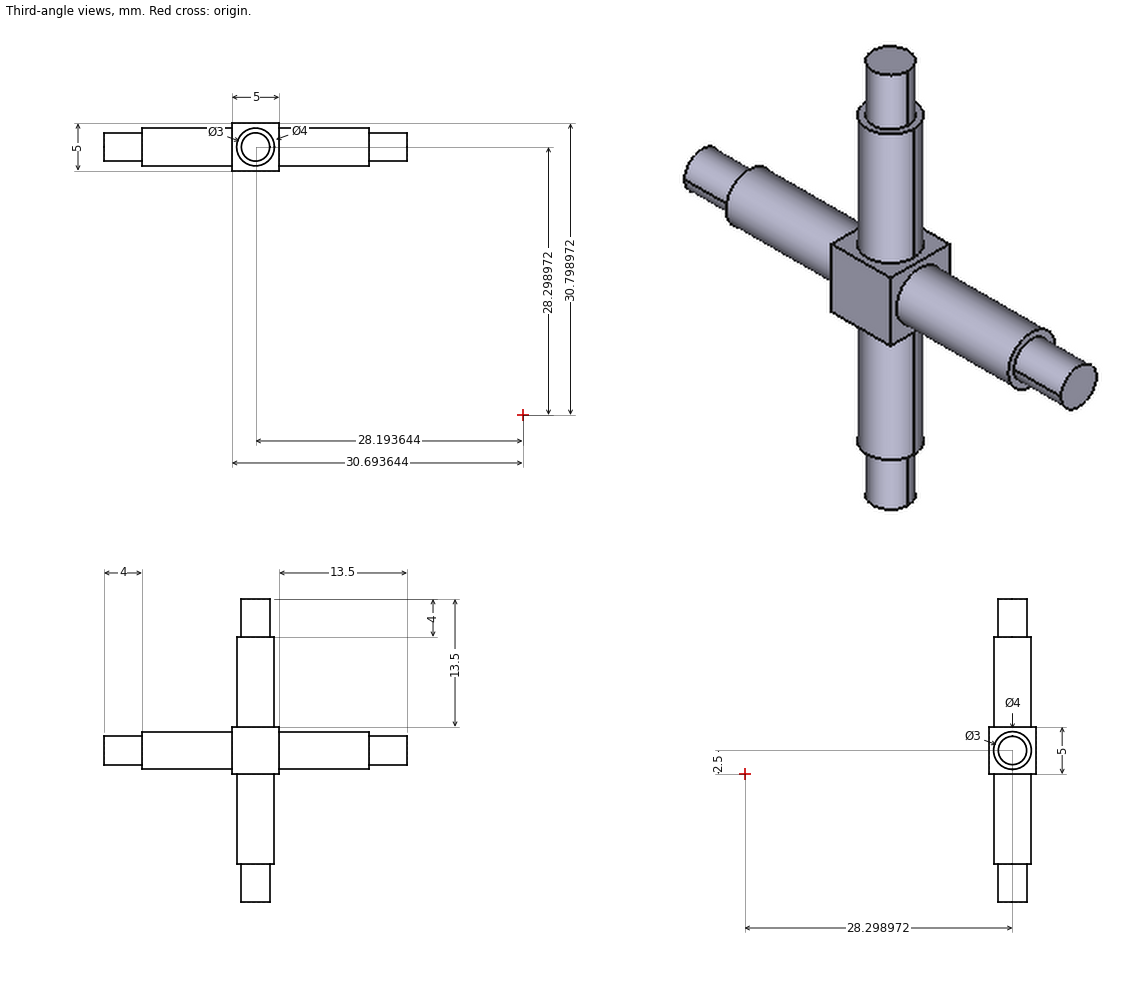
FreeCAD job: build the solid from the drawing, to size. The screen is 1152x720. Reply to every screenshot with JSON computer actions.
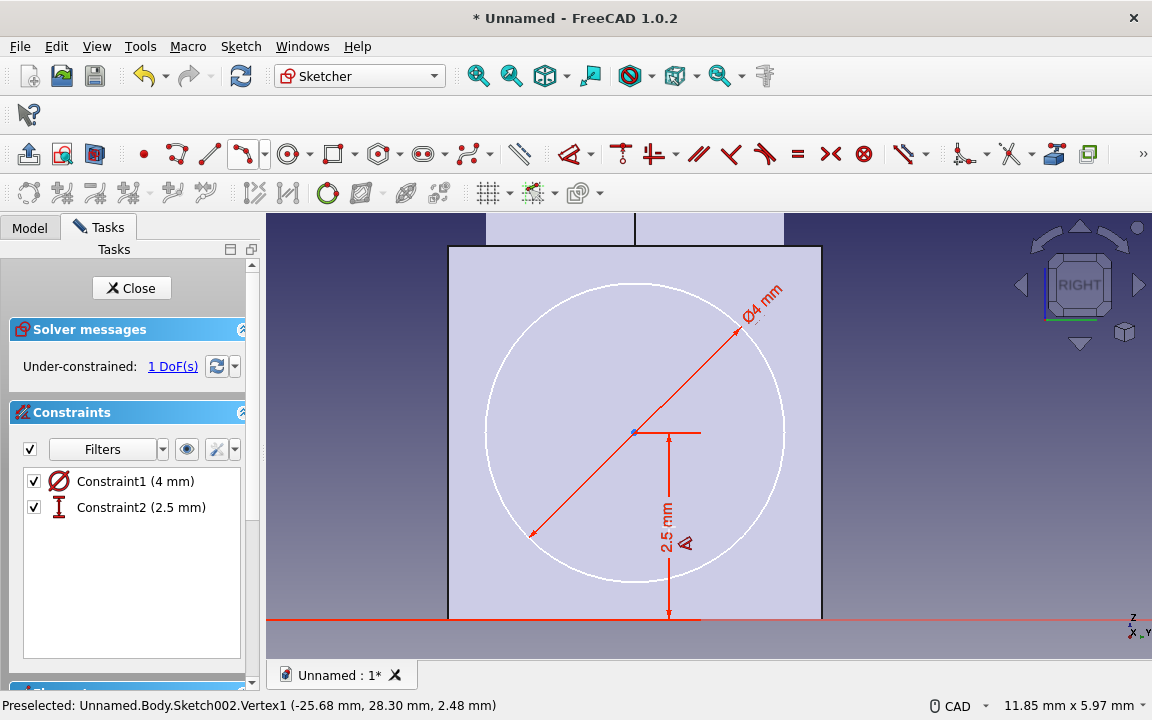
{"action": "left_click", "coordinate": [635, 433]}
{"action": "left_click", "coordinate": [464, 399]}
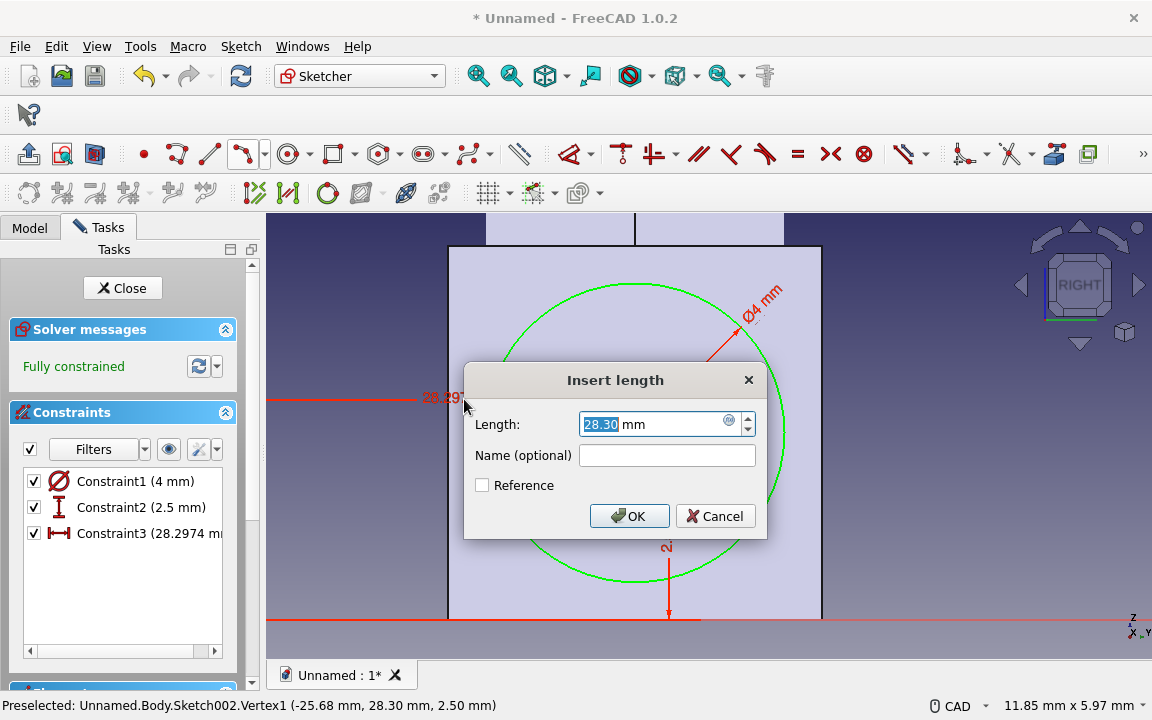
{"action": "type", "text": "28.298972"}
{"action": "key", "text": "Return"}
{"action": "key", "text": "Escape"}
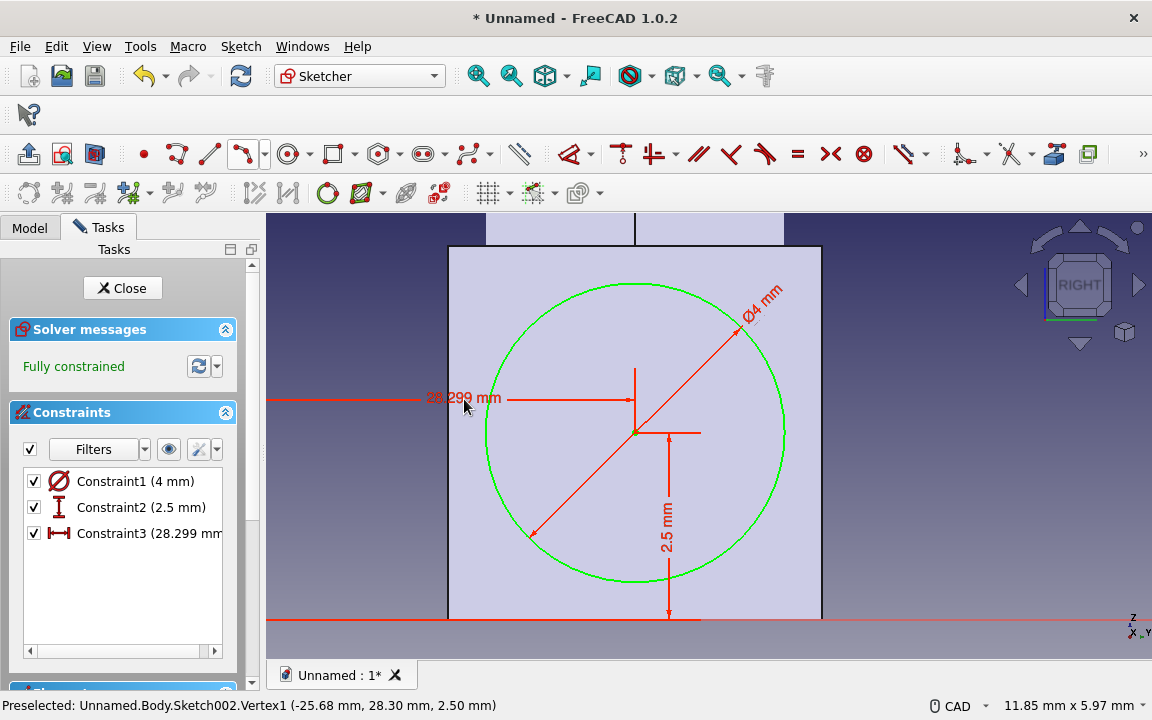
{"action": "left_click", "coordinate": [123, 288]}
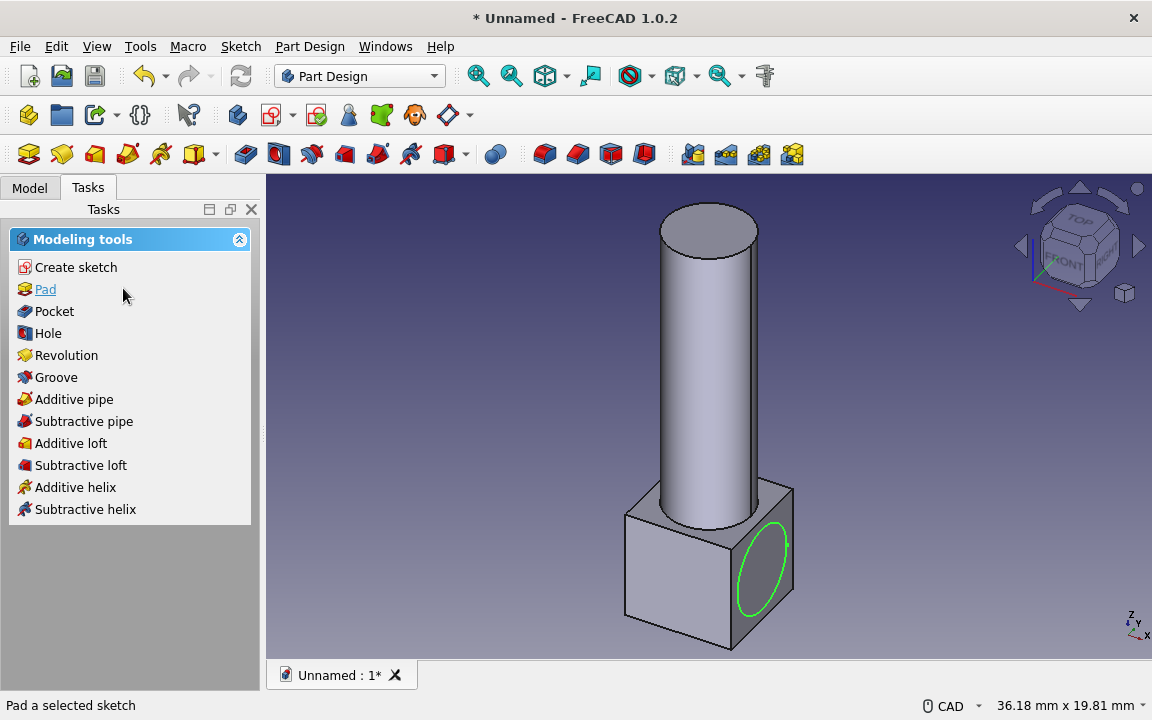
{"action": "left_click", "coordinate": [29, 154]}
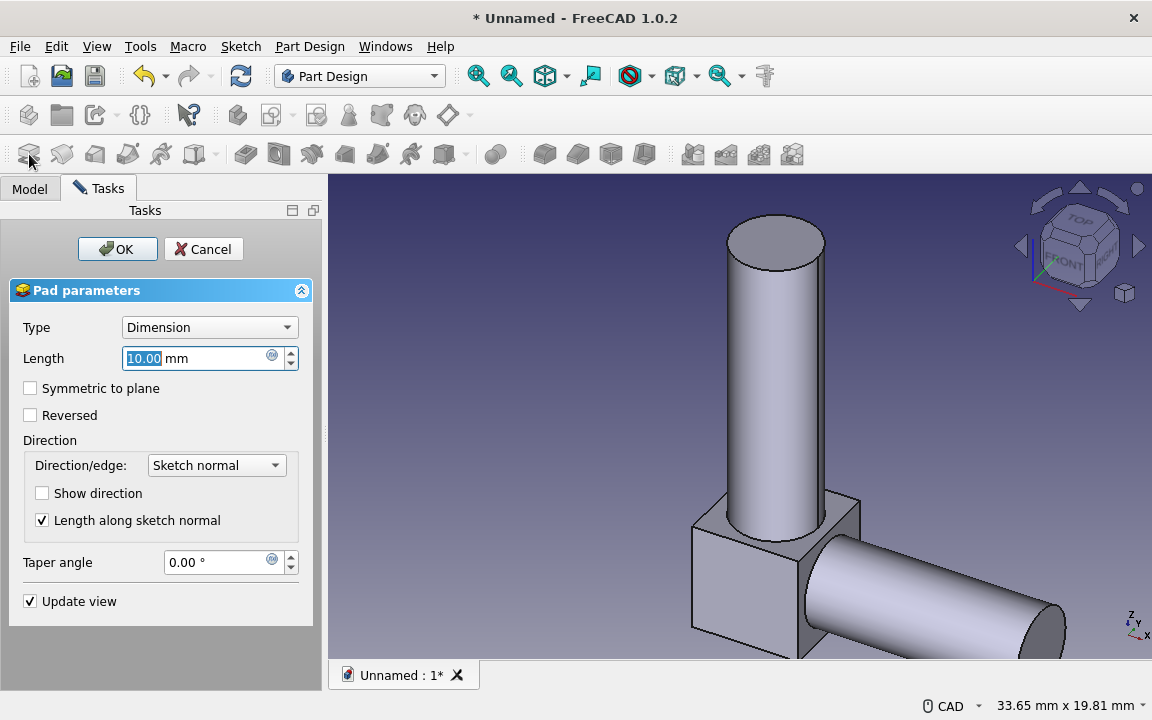
{"action": "type", "text": "13.5"}
{"action": "key", "text": "Tab"}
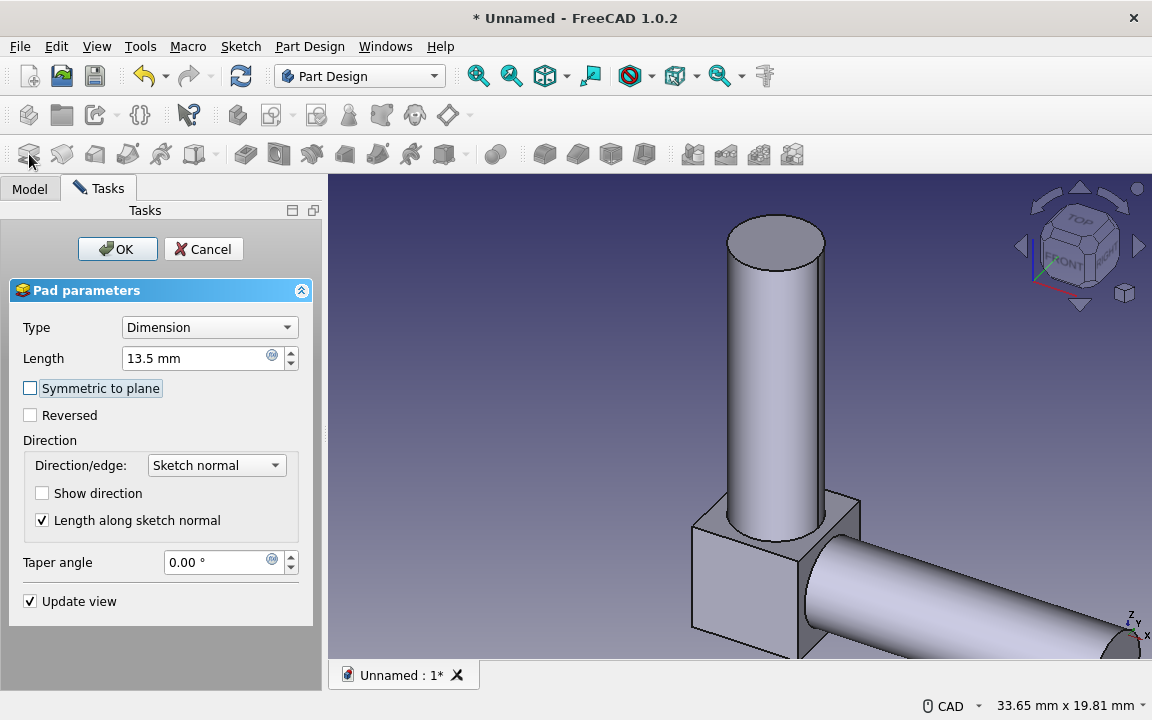
{"action": "left_click", "coordinate": [118, 249]}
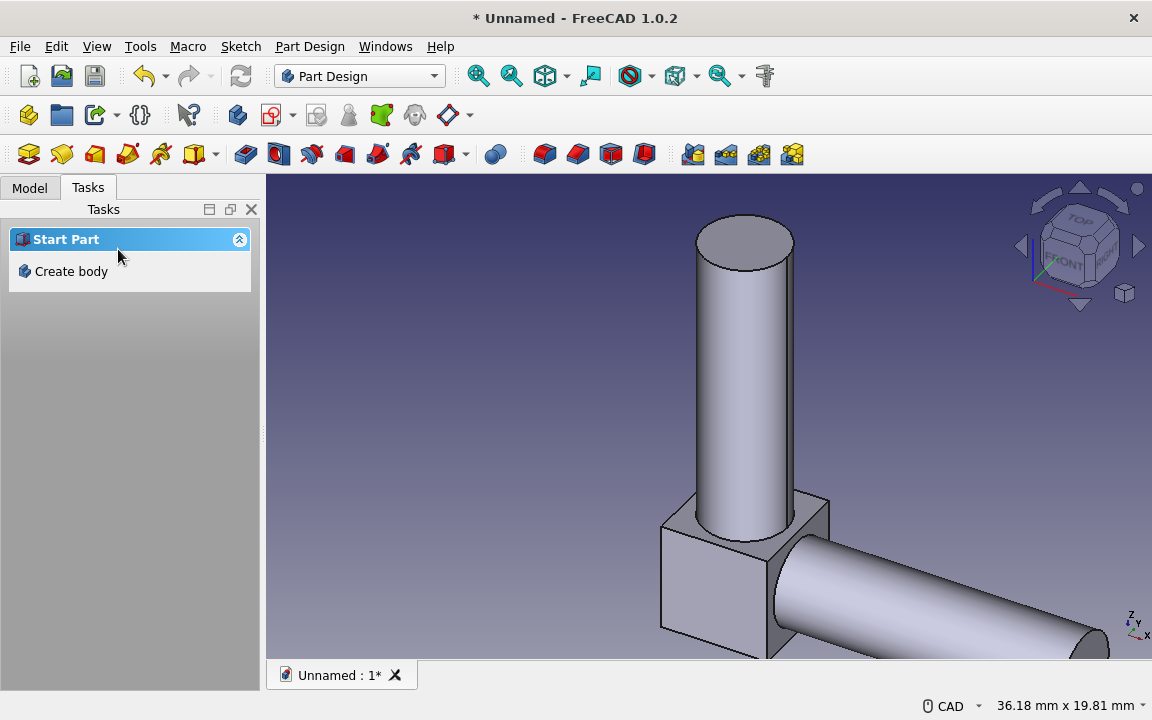
{"action": "key", "text": "v f"}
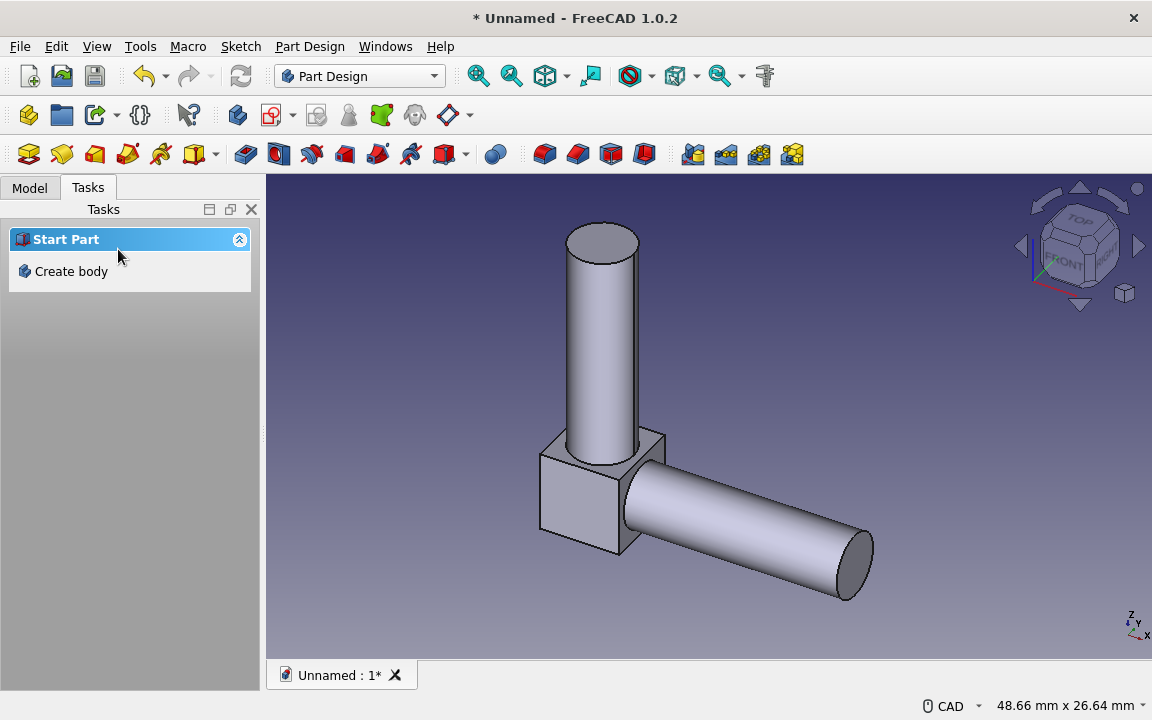
{"action": "left_click", "coordinate": [30, 188]}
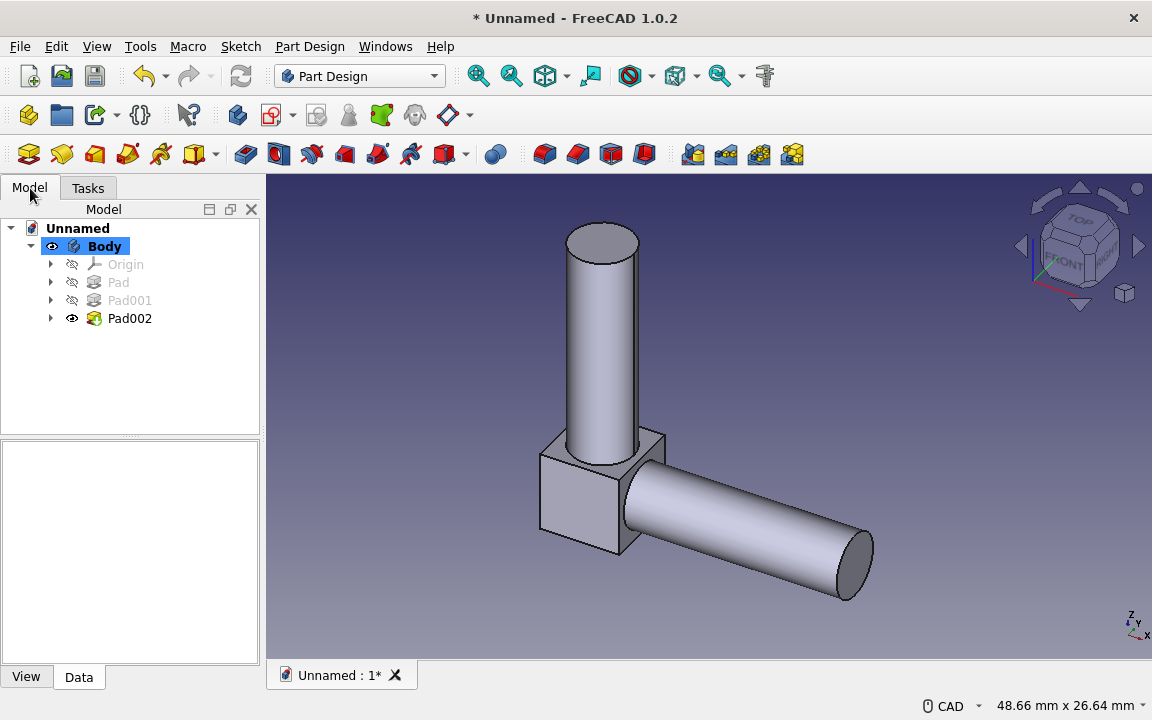
{"action": "left_click", "coordinate": [51, 264]}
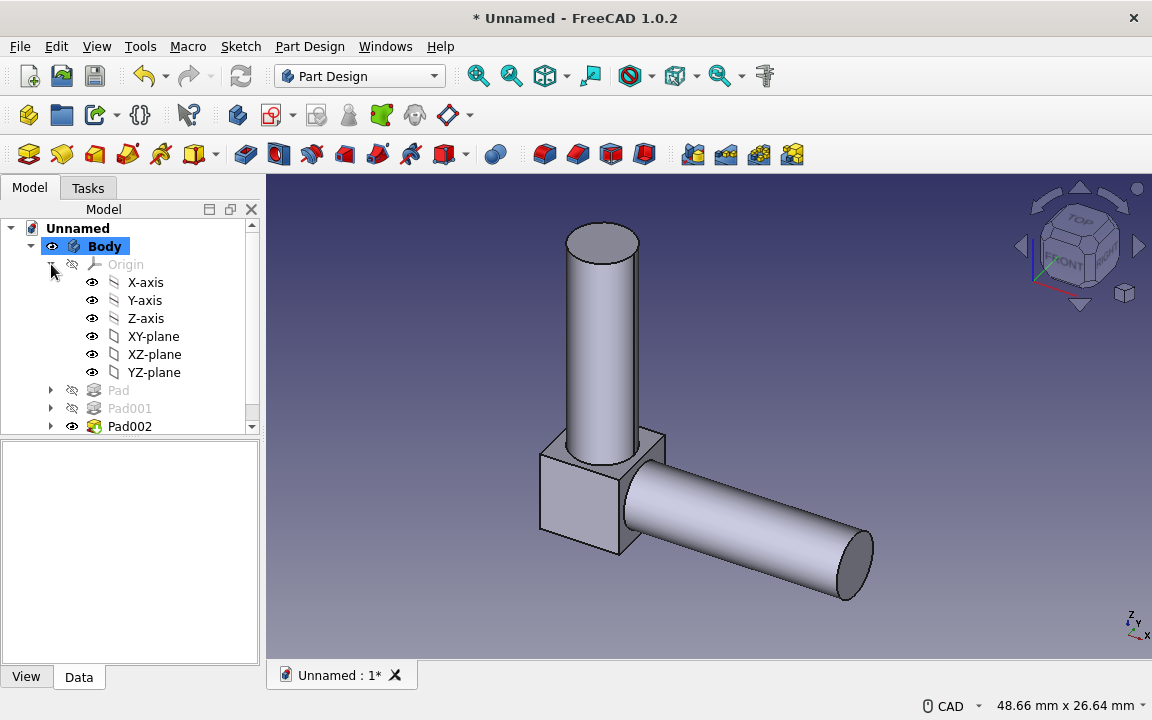
{"action": "left_click", "coordinate": [137, 336]}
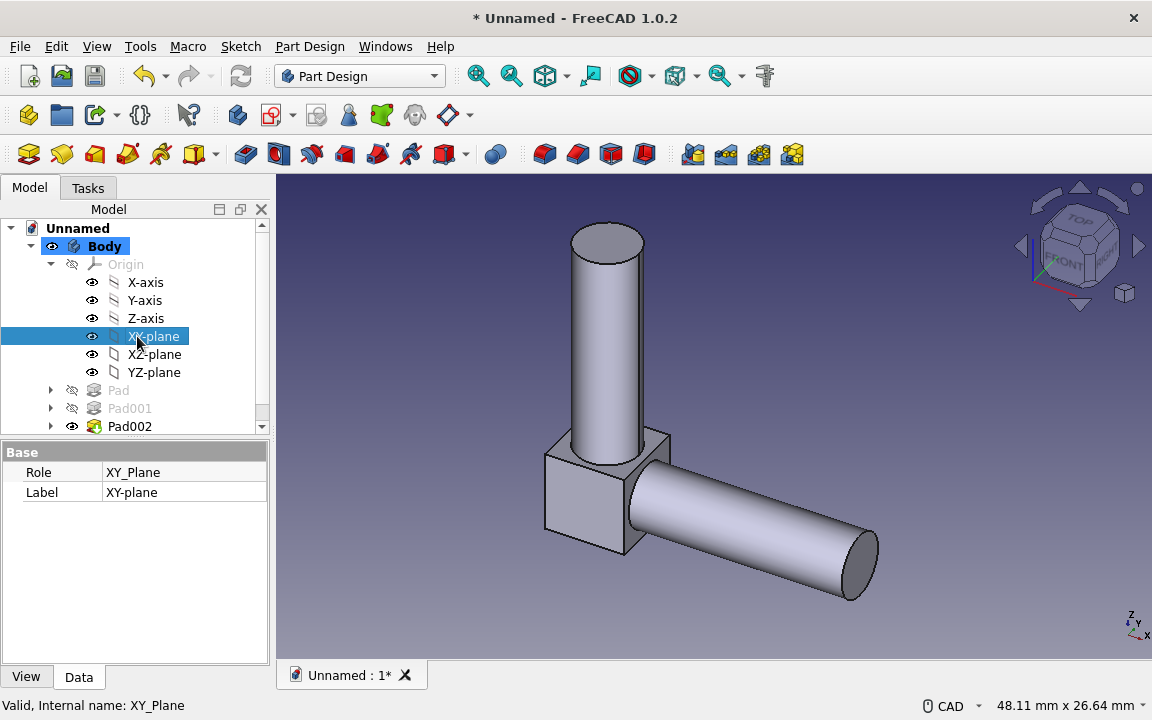
{"action": "left_click", "coordinate": [448, 116]}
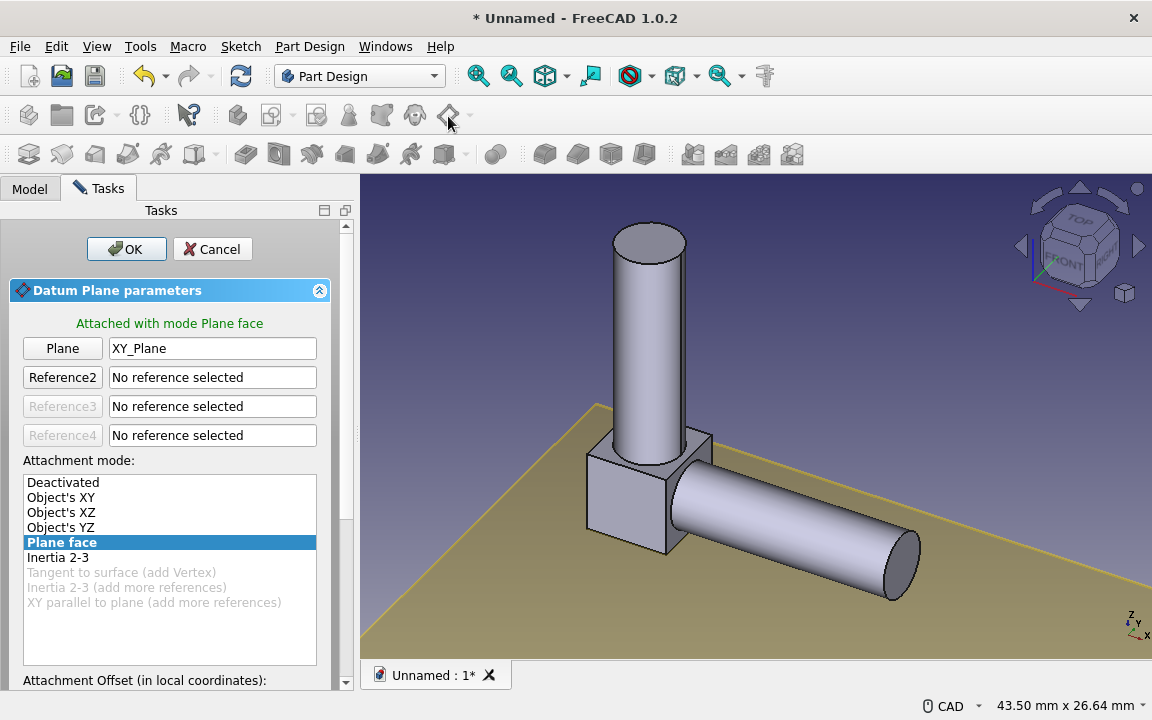
{"action": "scroll", "coordinate": [346, 455], "scroll_direction": "down", "scroll_amount": 3}